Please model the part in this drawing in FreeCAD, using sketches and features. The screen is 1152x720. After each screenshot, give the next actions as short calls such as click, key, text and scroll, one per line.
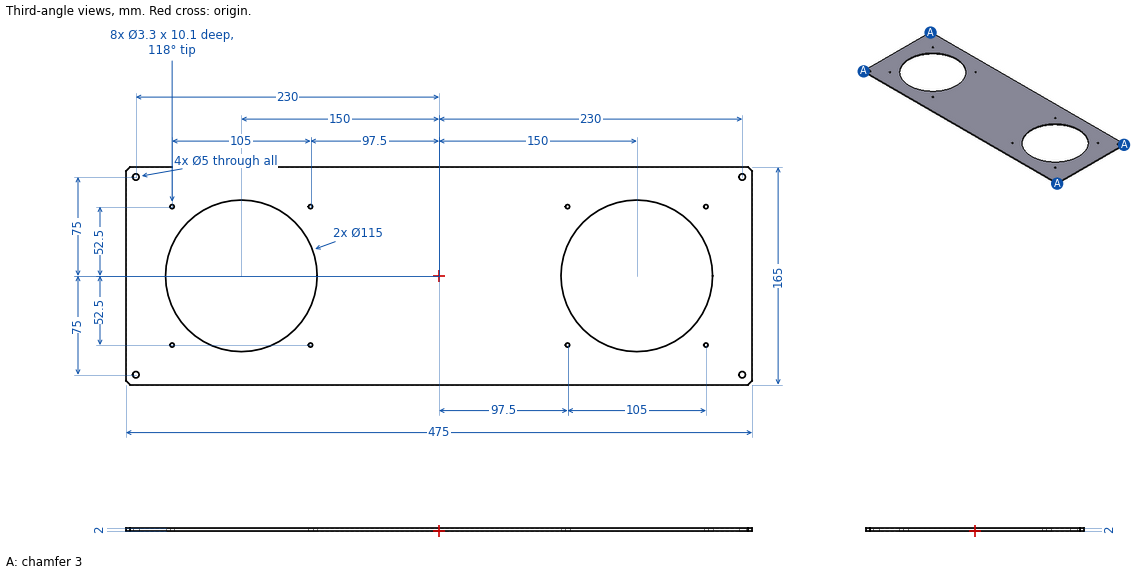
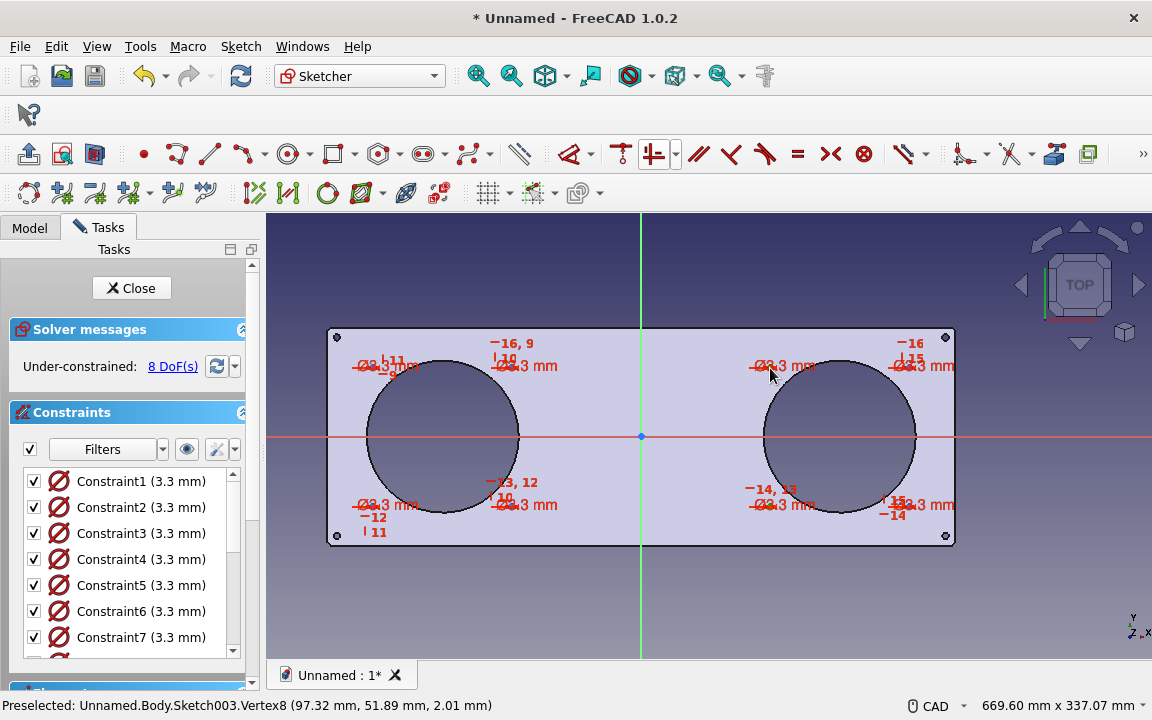
key(v)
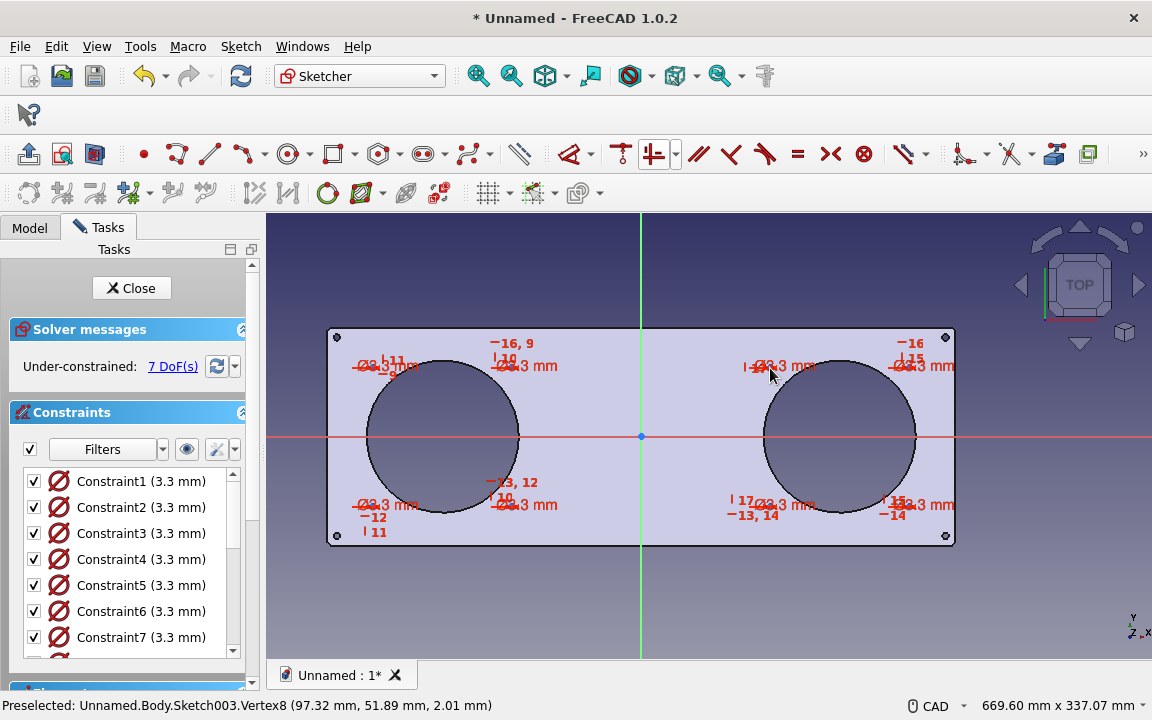
click(909, 368)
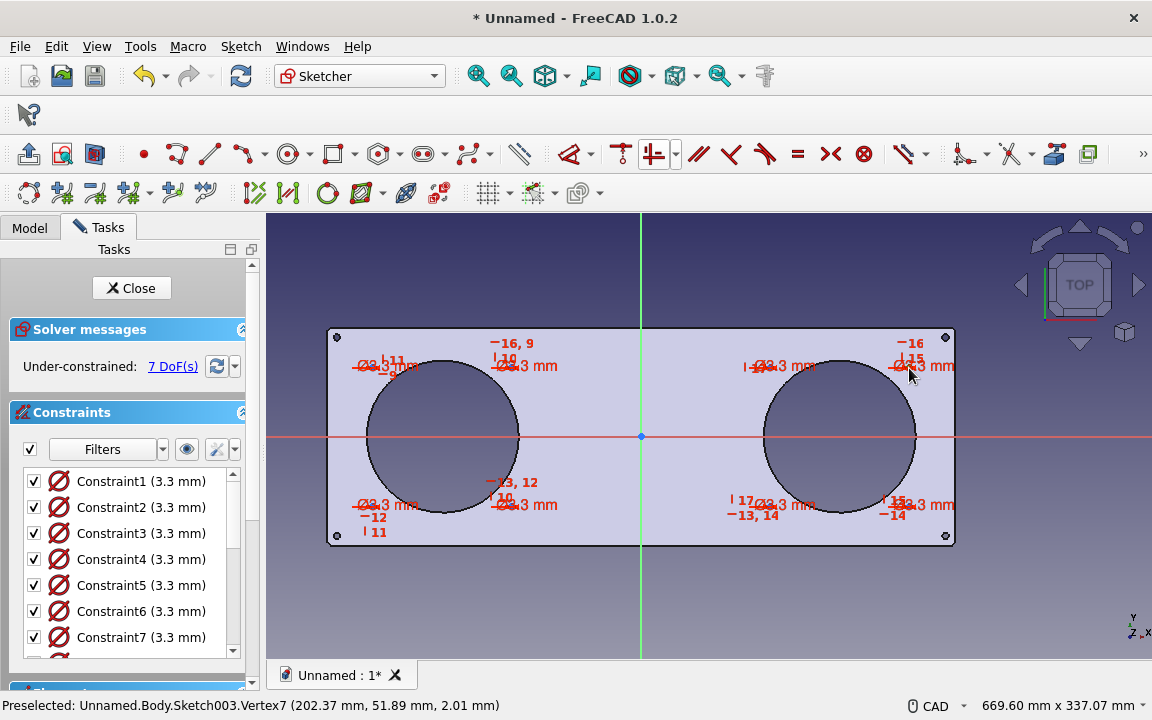
click(770, 368)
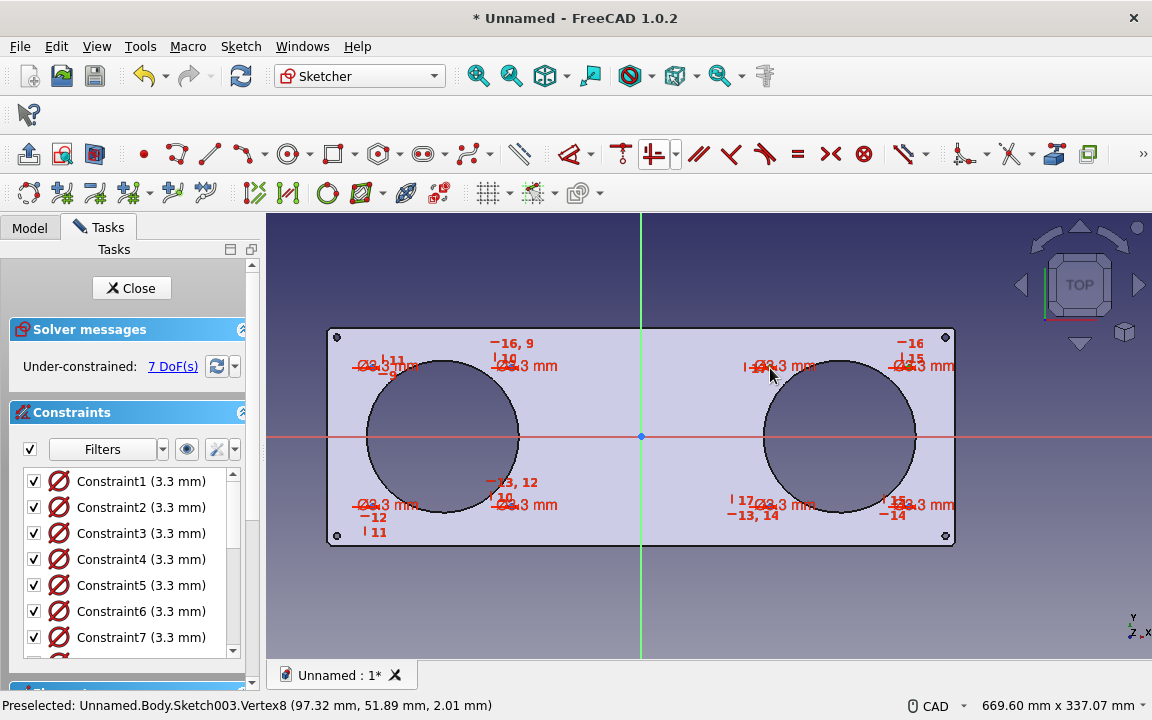
key(h)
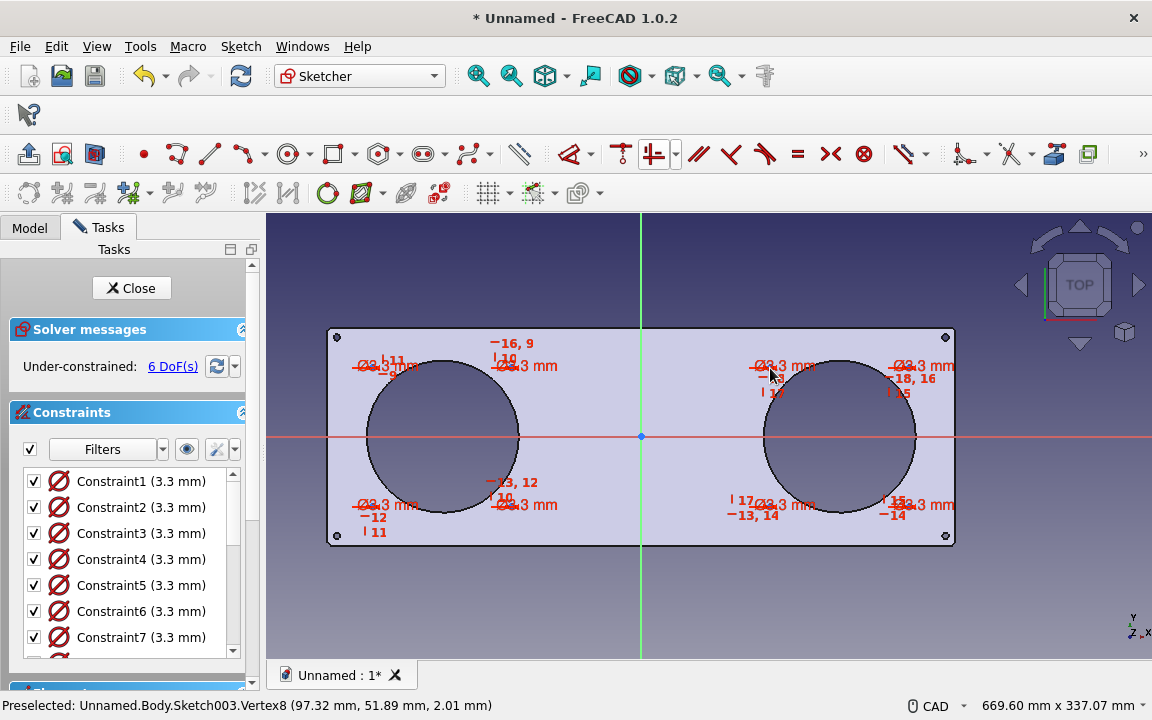
key(d)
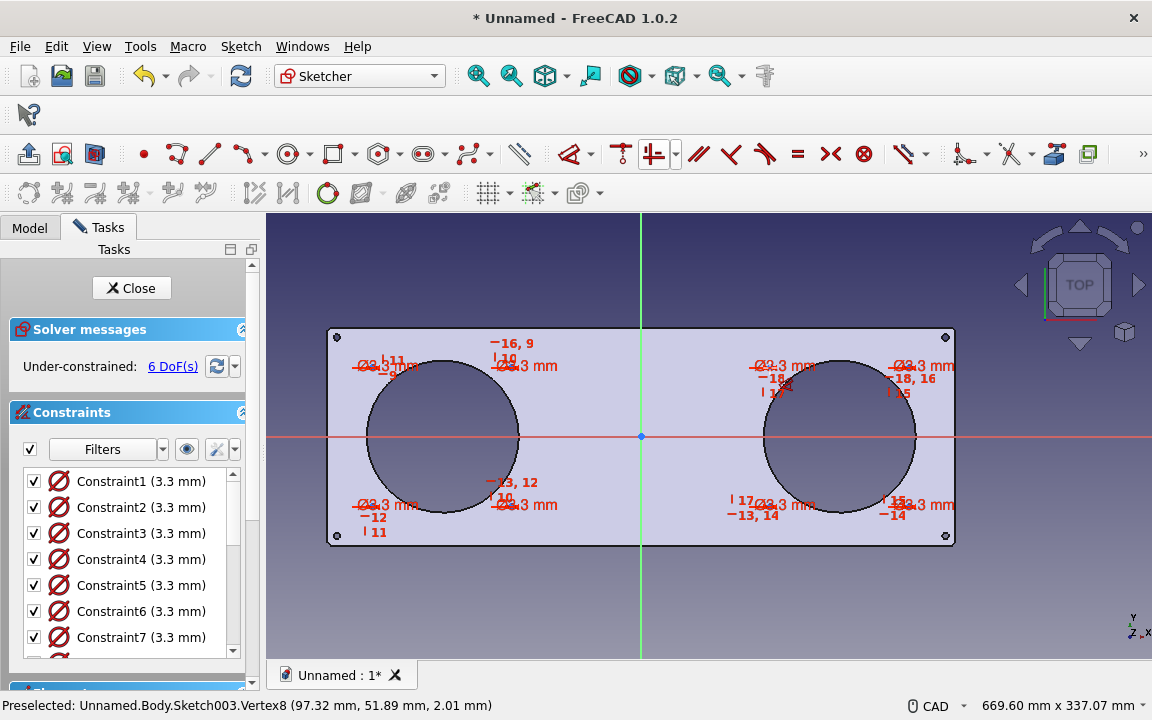
click(373, 368)
click(339, 402)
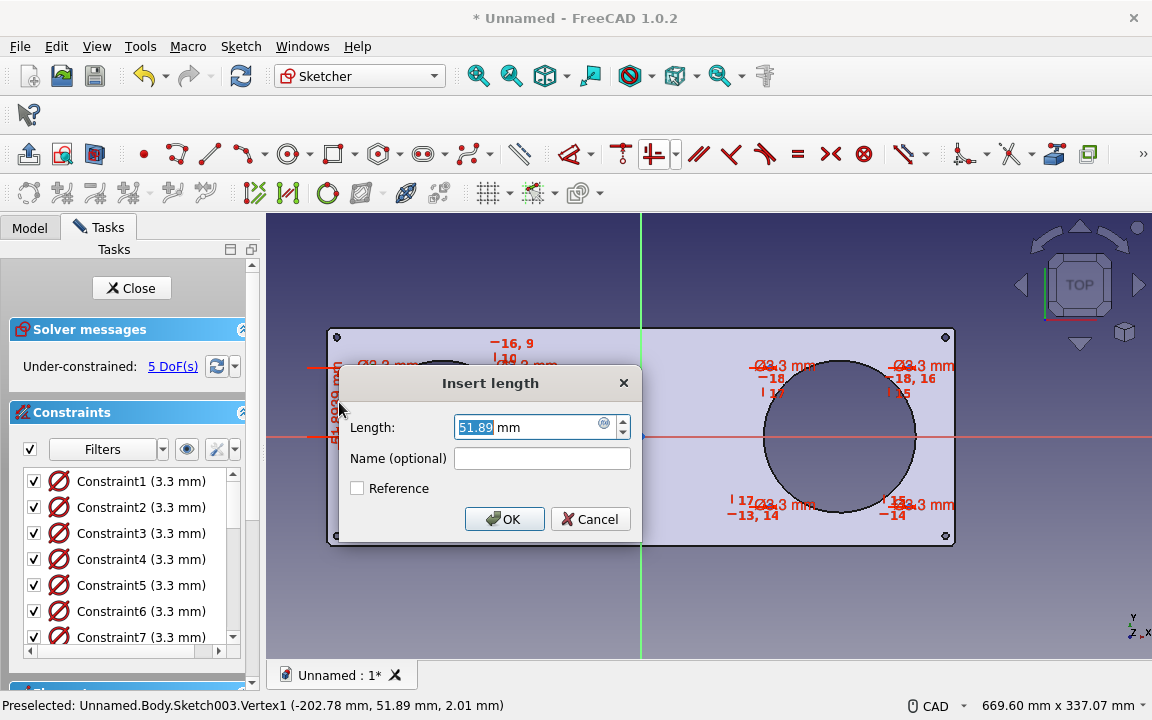
text(52.5)
key(Return)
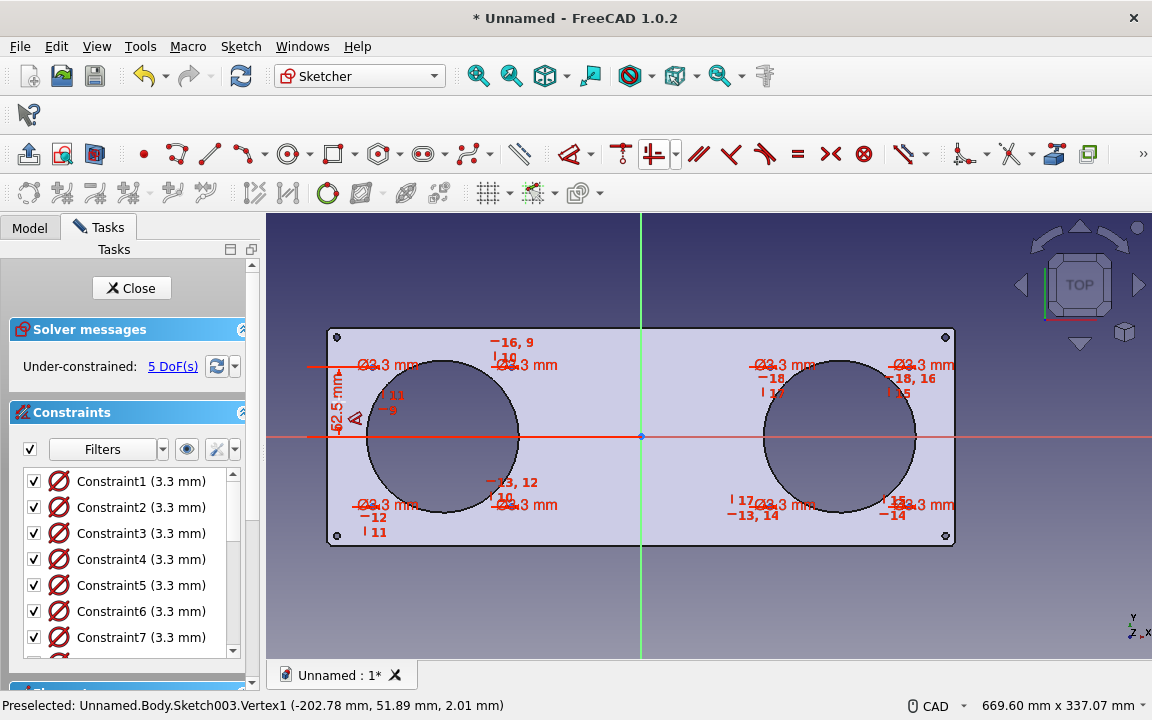
click(512, 367)
click(577, 333)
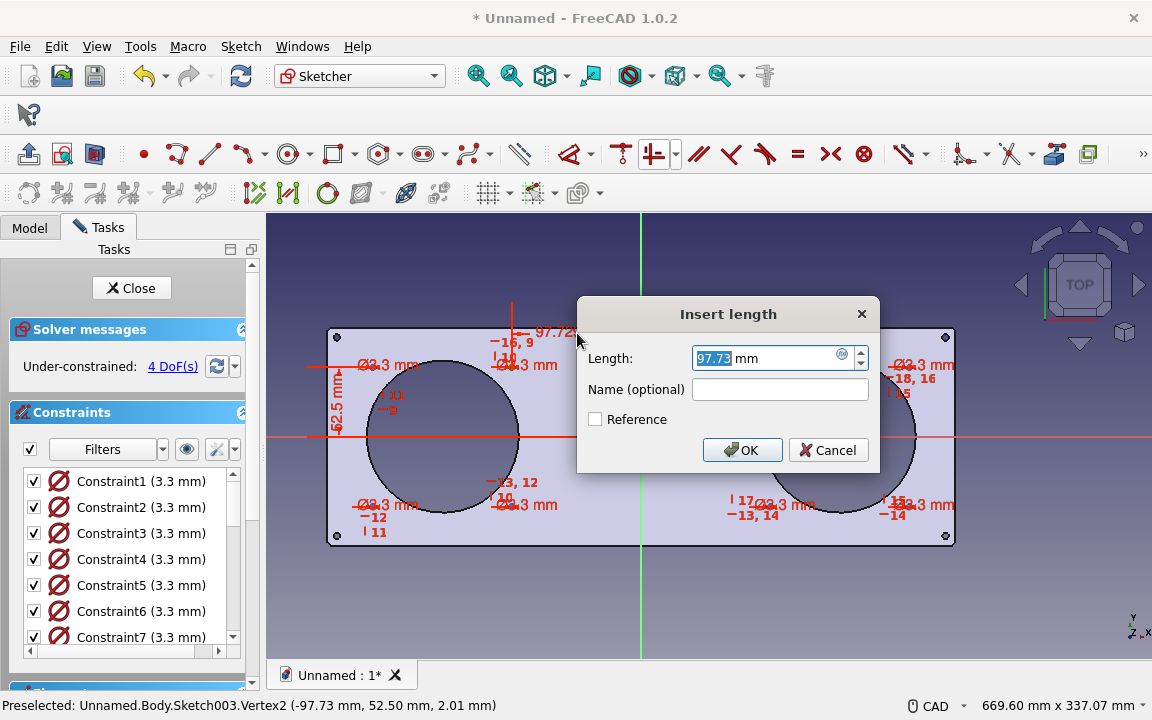
text(97.5)
key(Return)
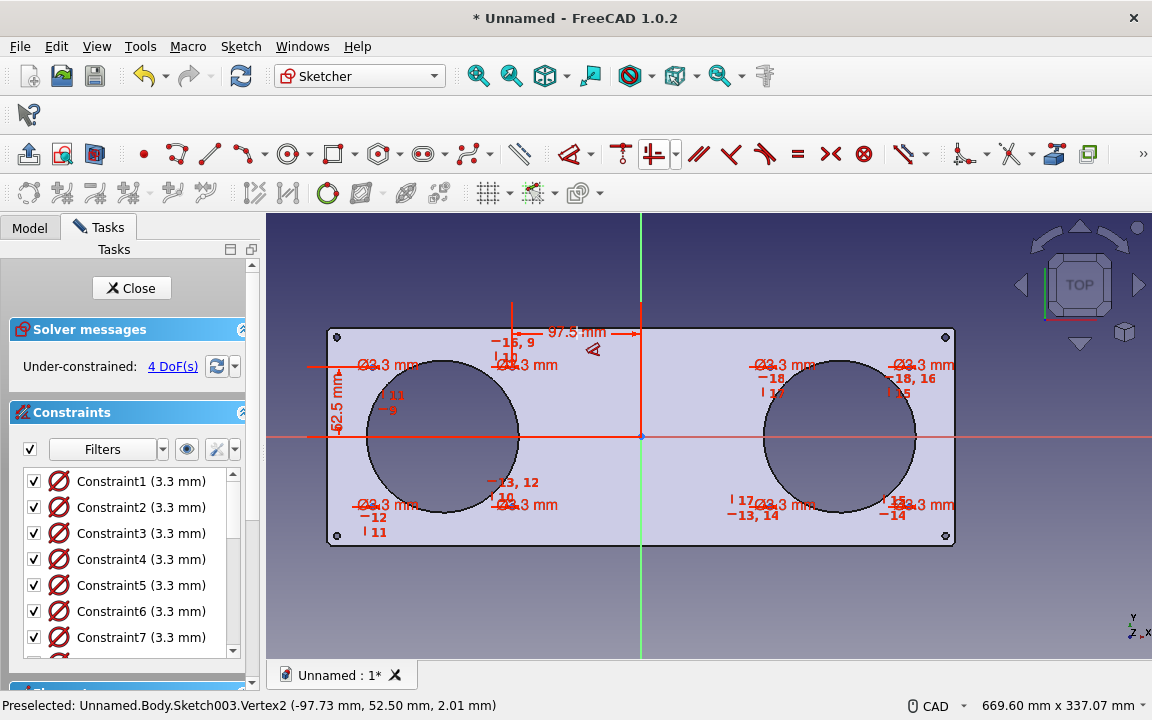
click(512, 507)
click(478, 472)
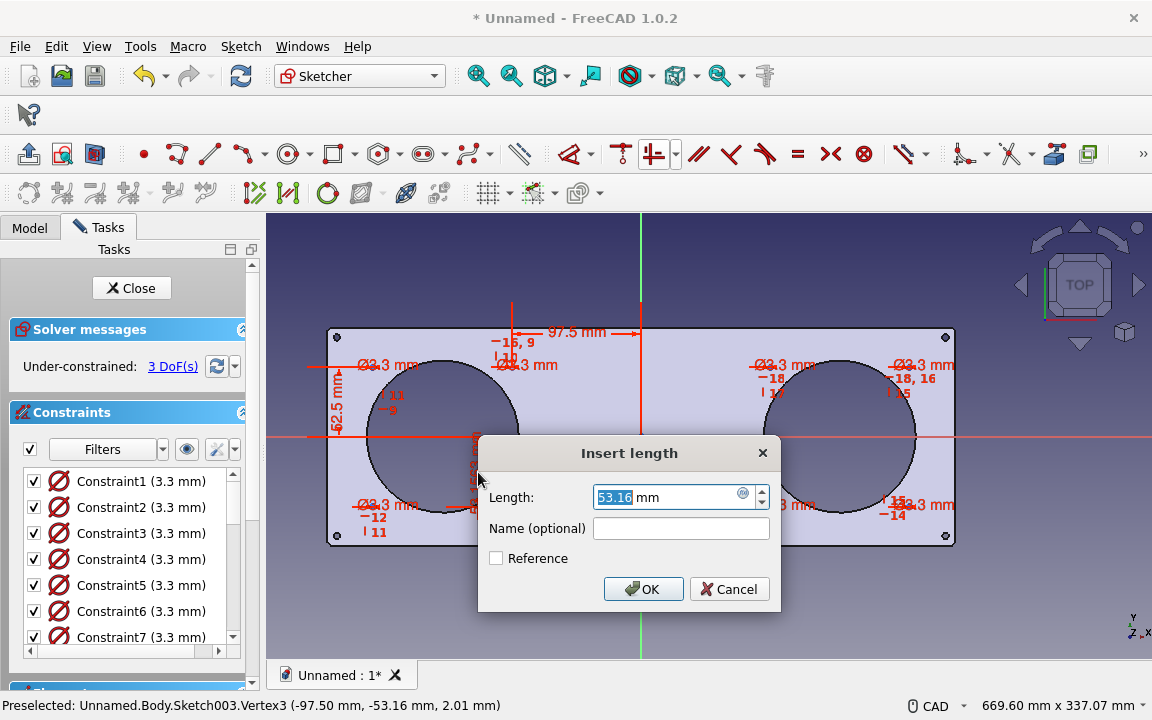
text(52.5)
key(Return)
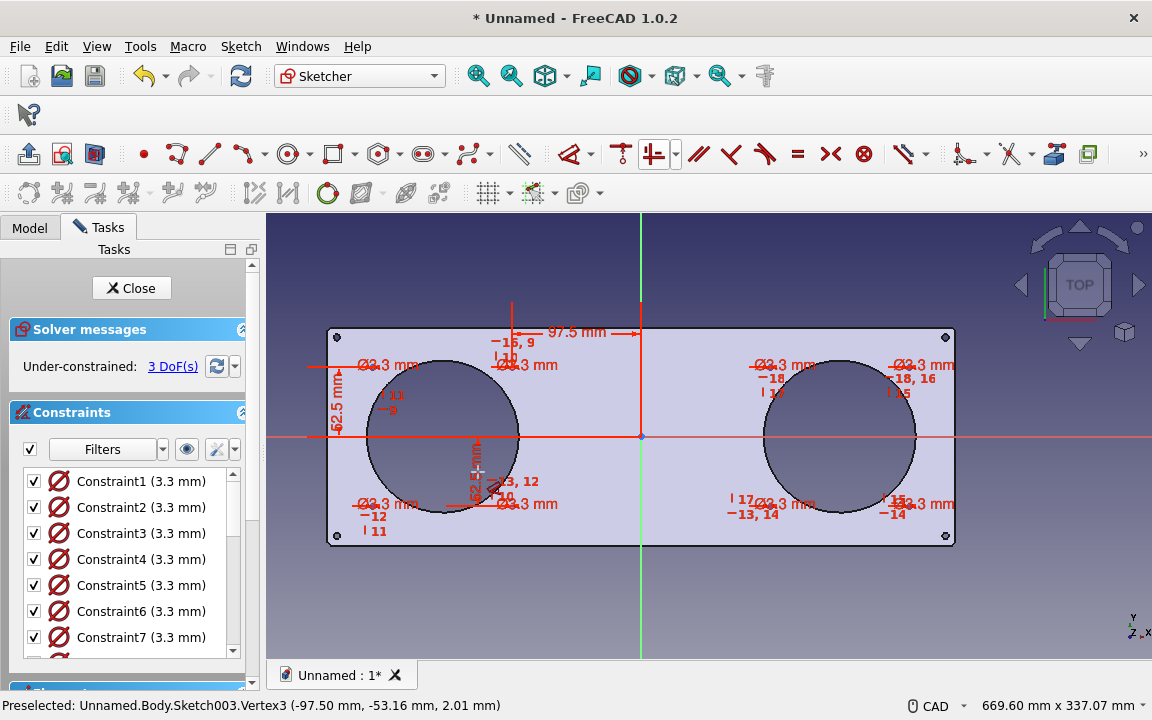
click(770, 506)
click(706, 540)